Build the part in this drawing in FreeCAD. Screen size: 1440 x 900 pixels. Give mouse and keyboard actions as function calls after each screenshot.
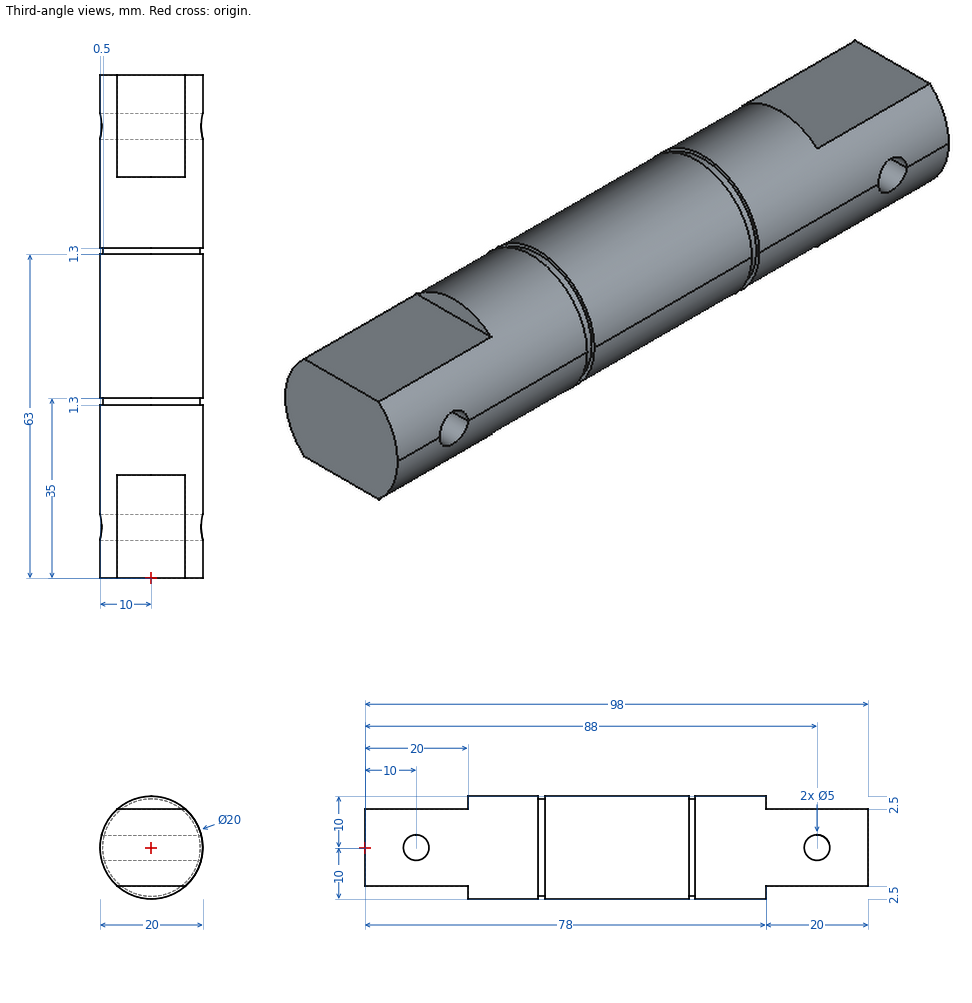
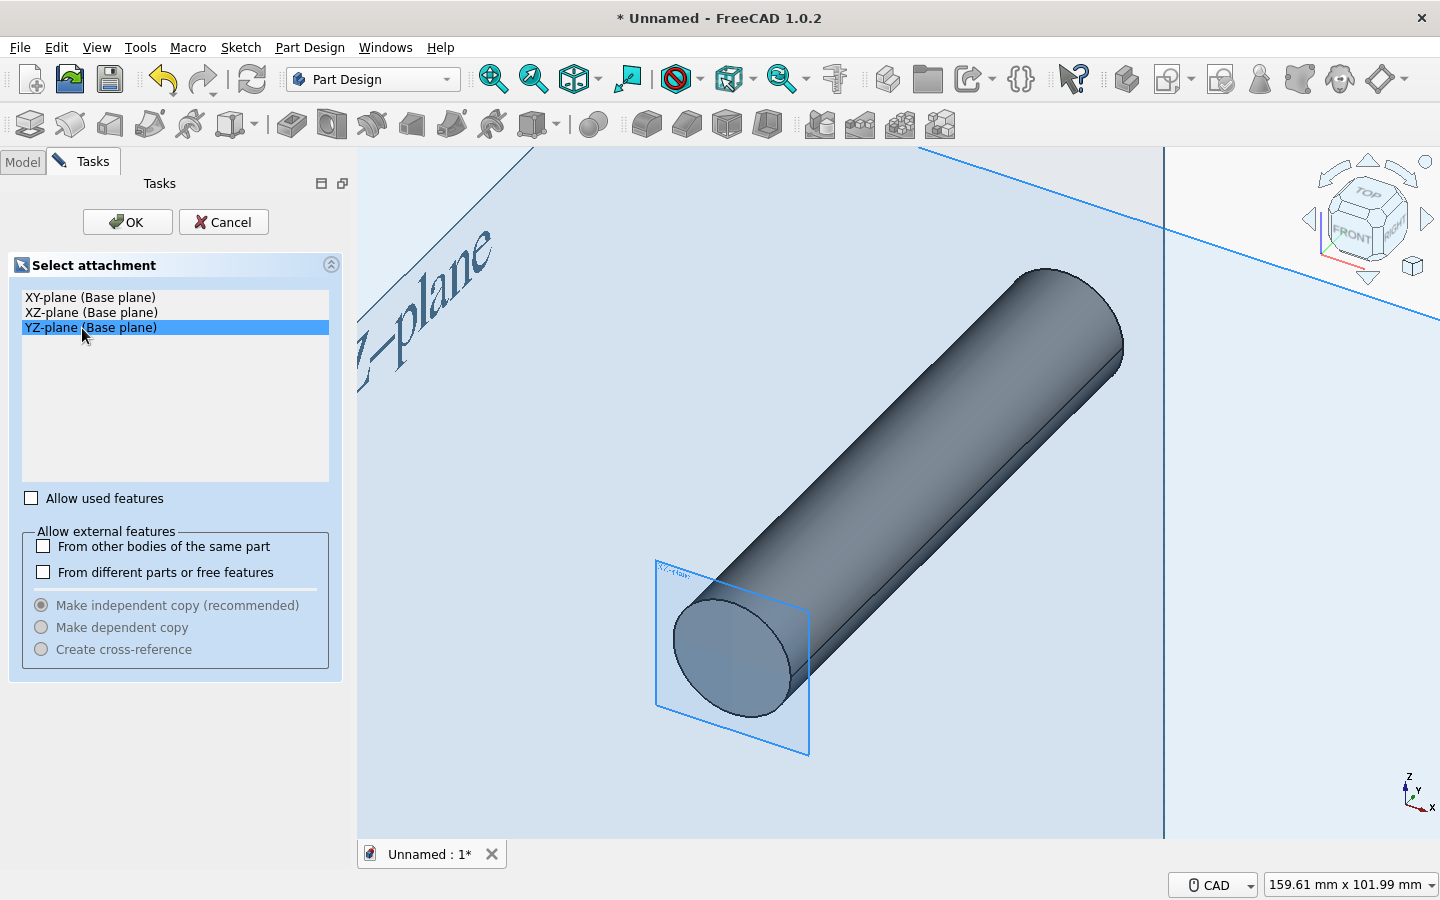
click(128, 222)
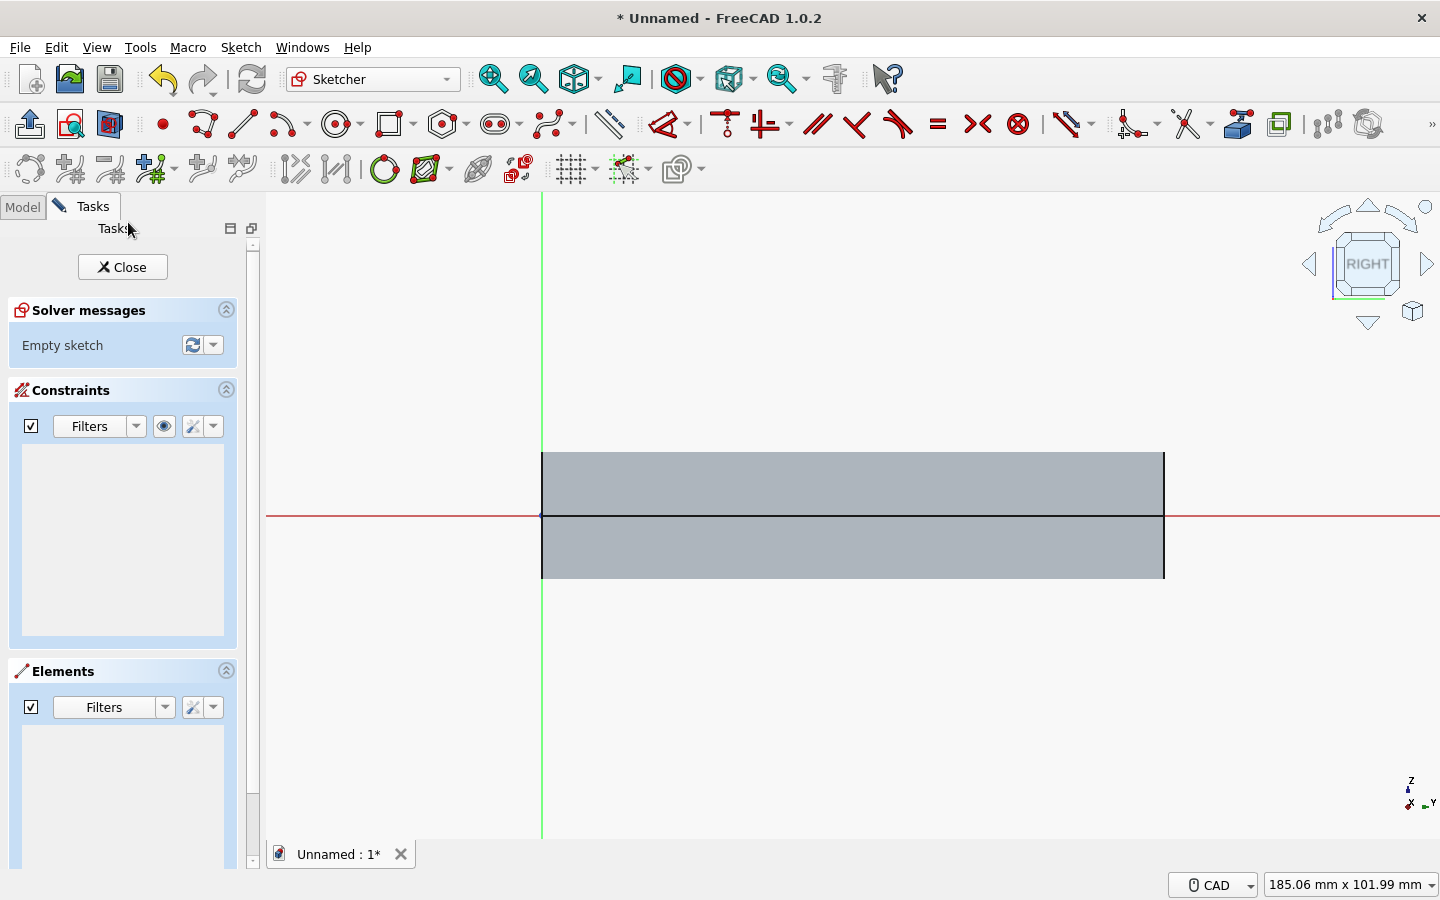
click(110, 124)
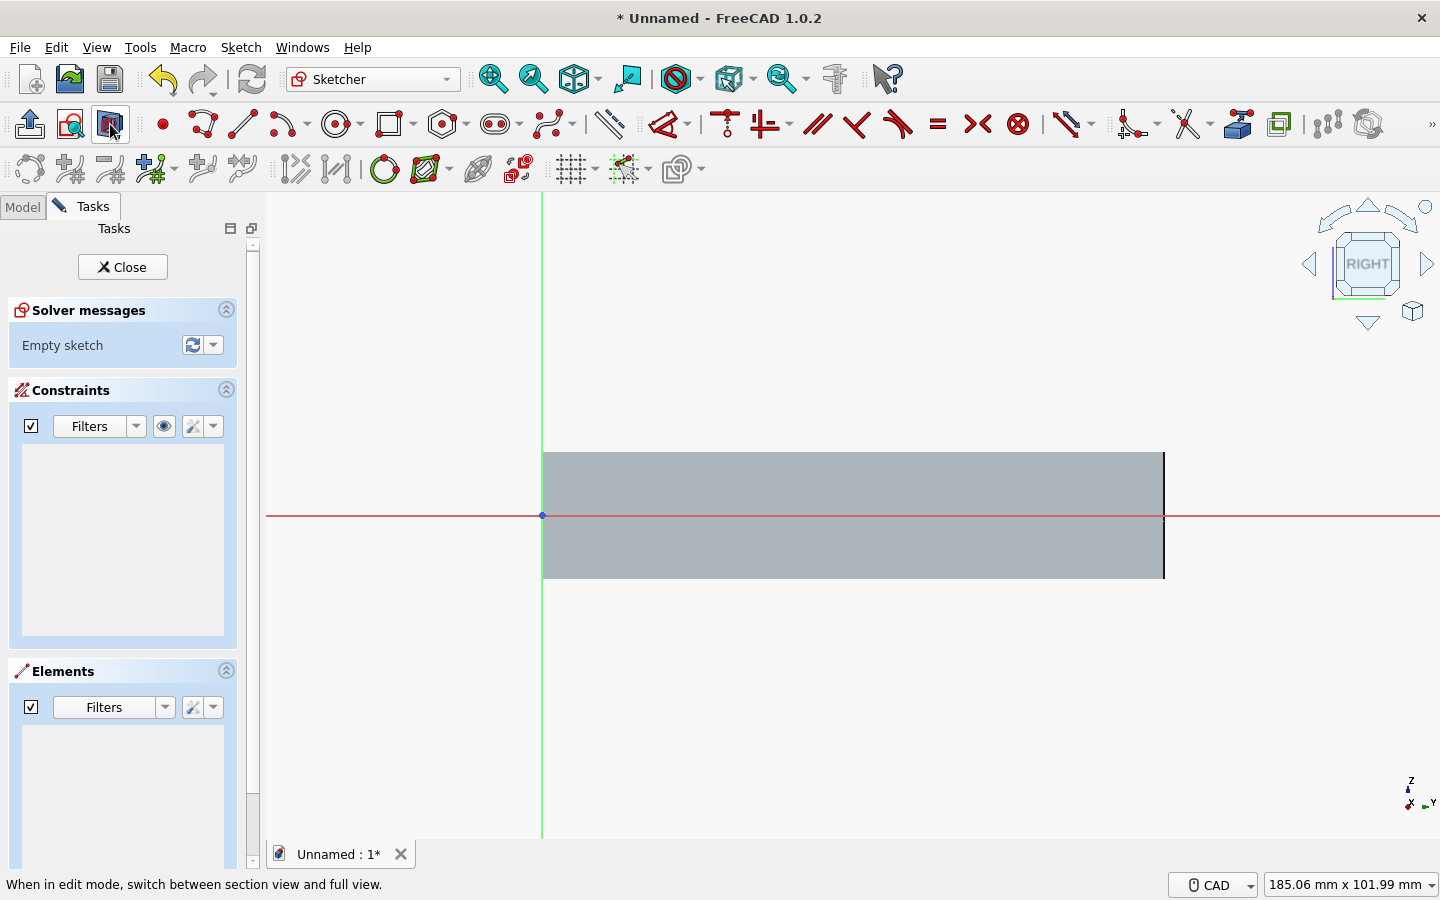
key(g)
key(r)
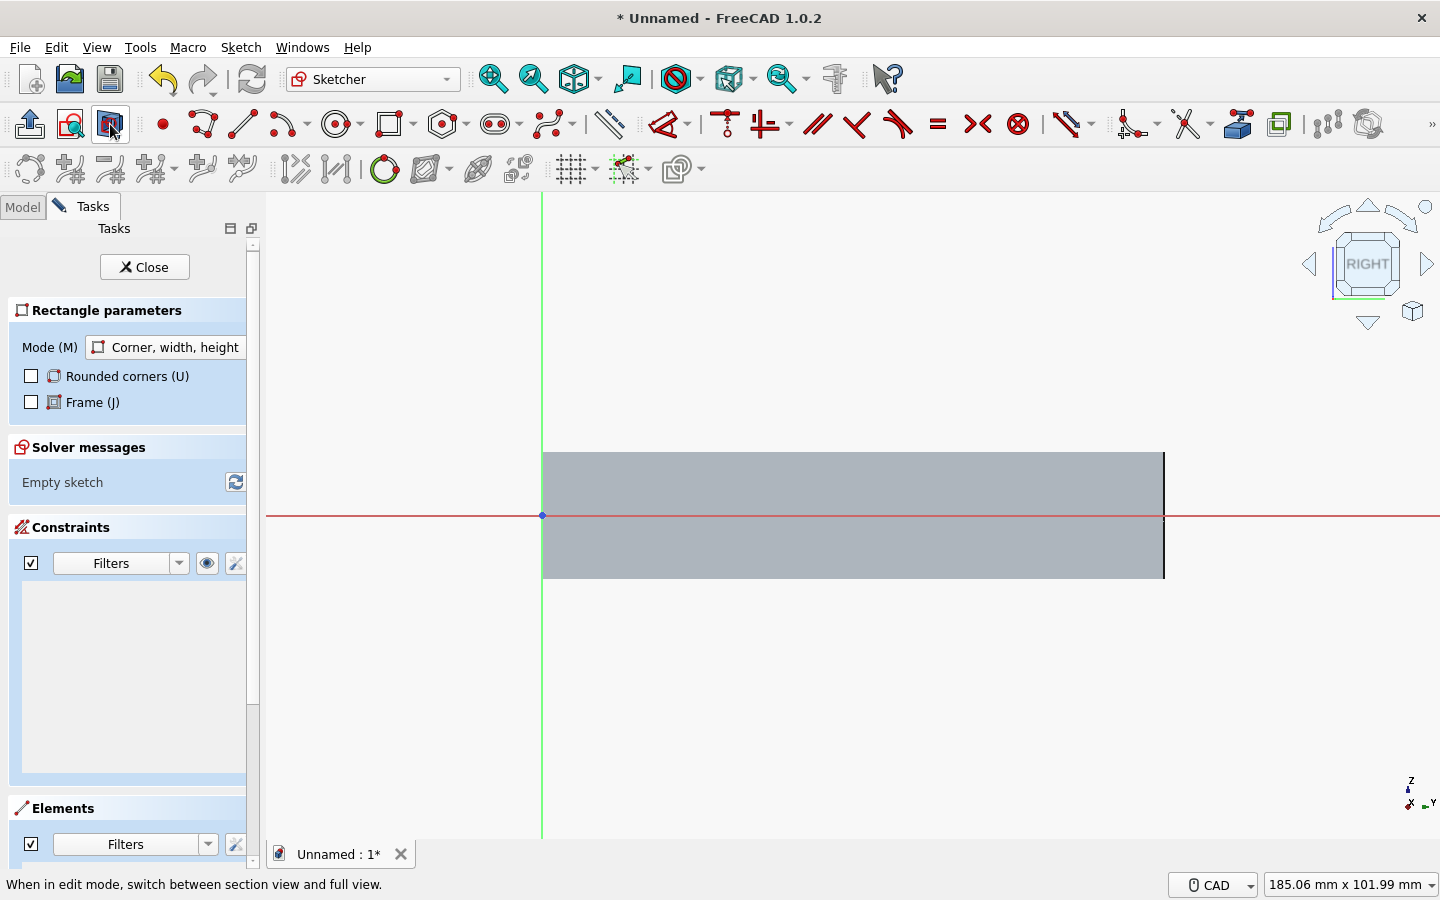
click(1037, 563)
move(1164, 579)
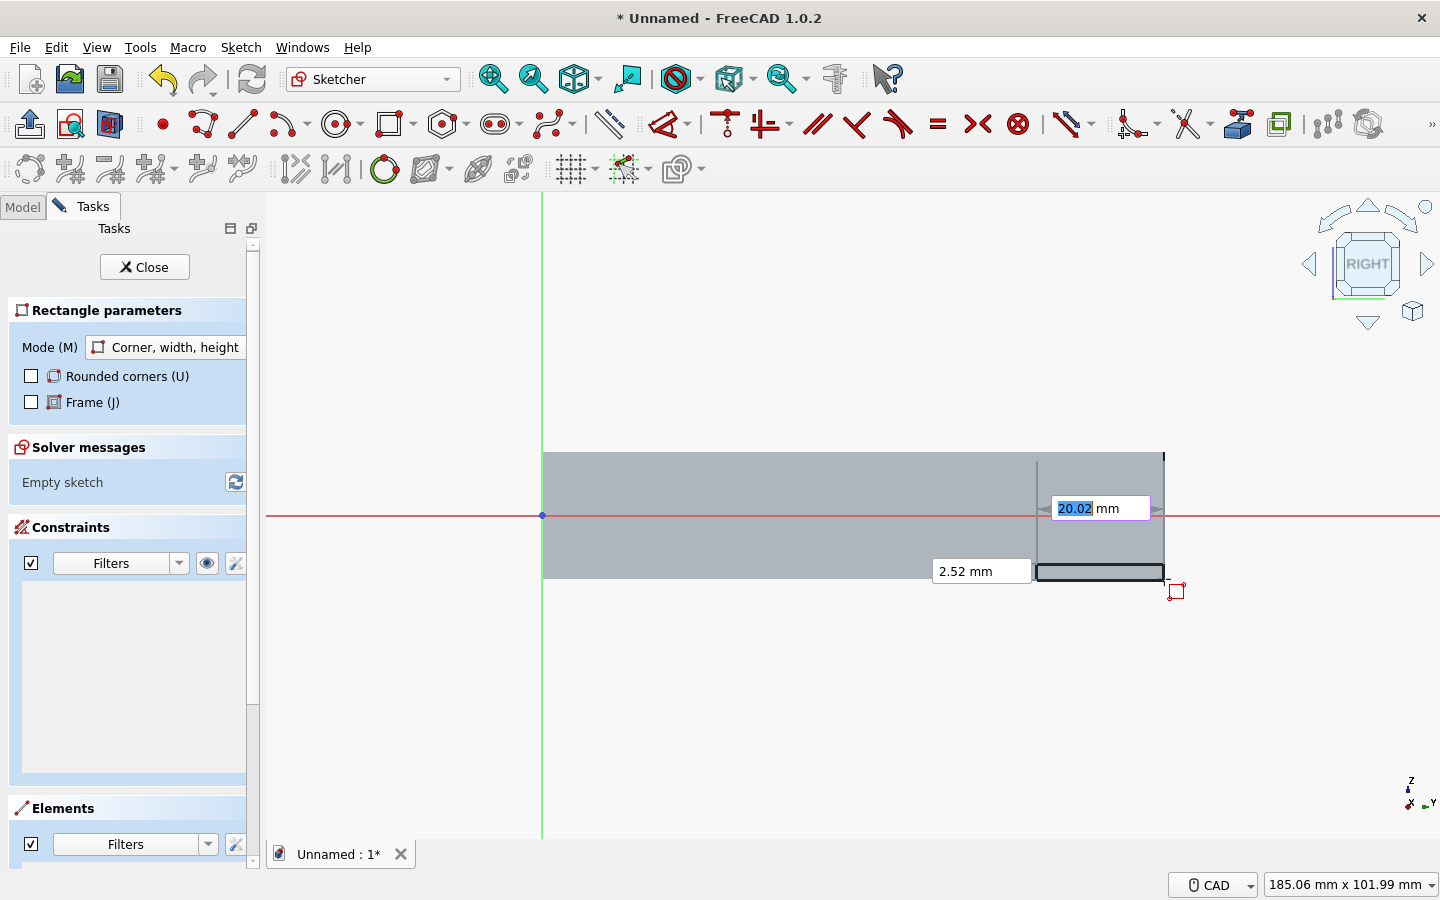
text(20)
key(Tab)
text(2.5)
key(Return)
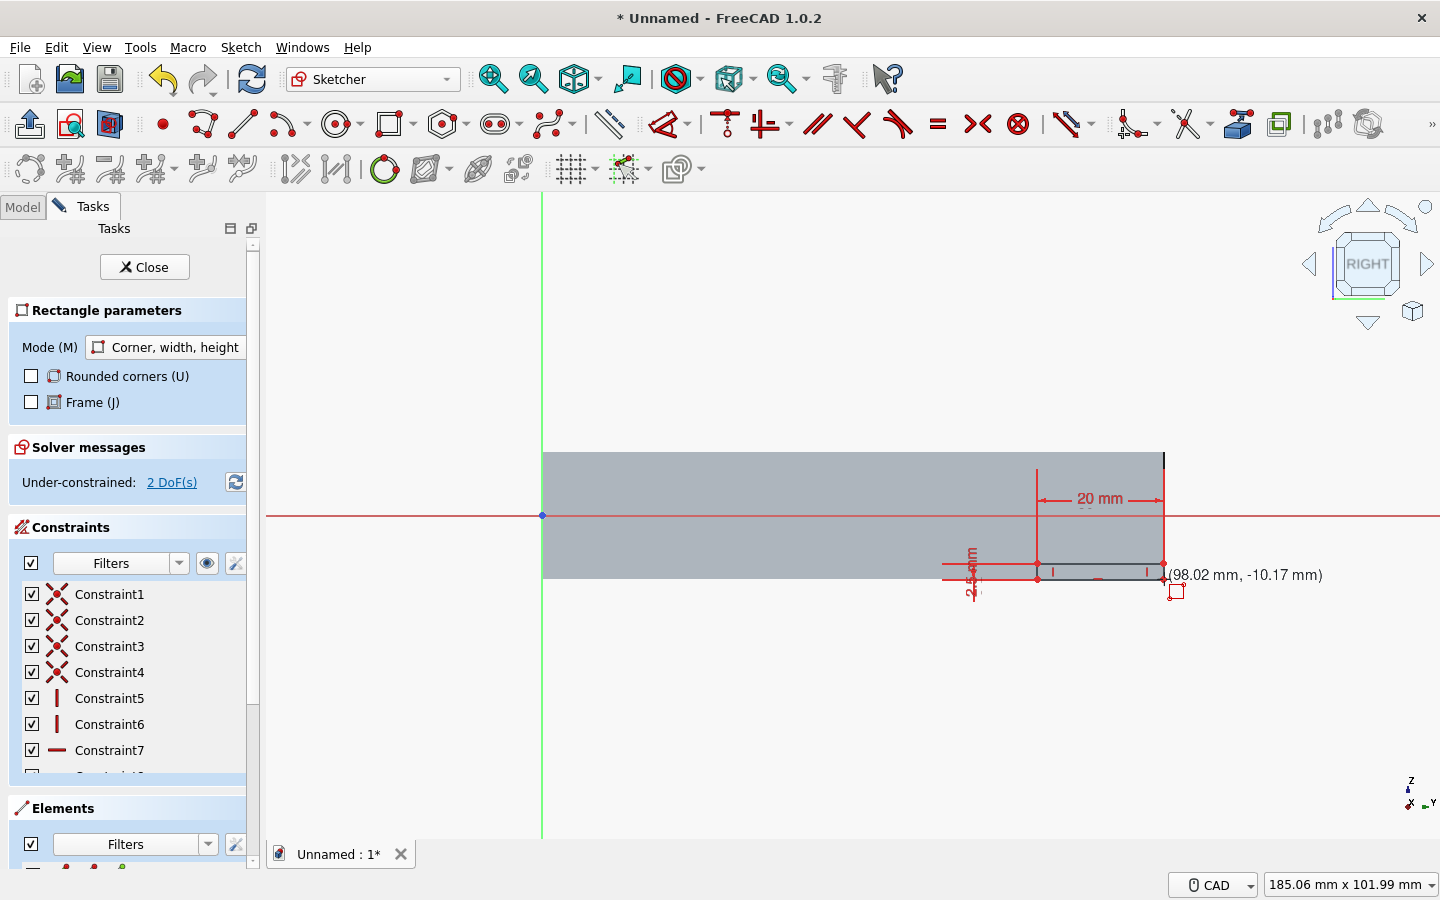
click(1037, 452)
move(1164, 468)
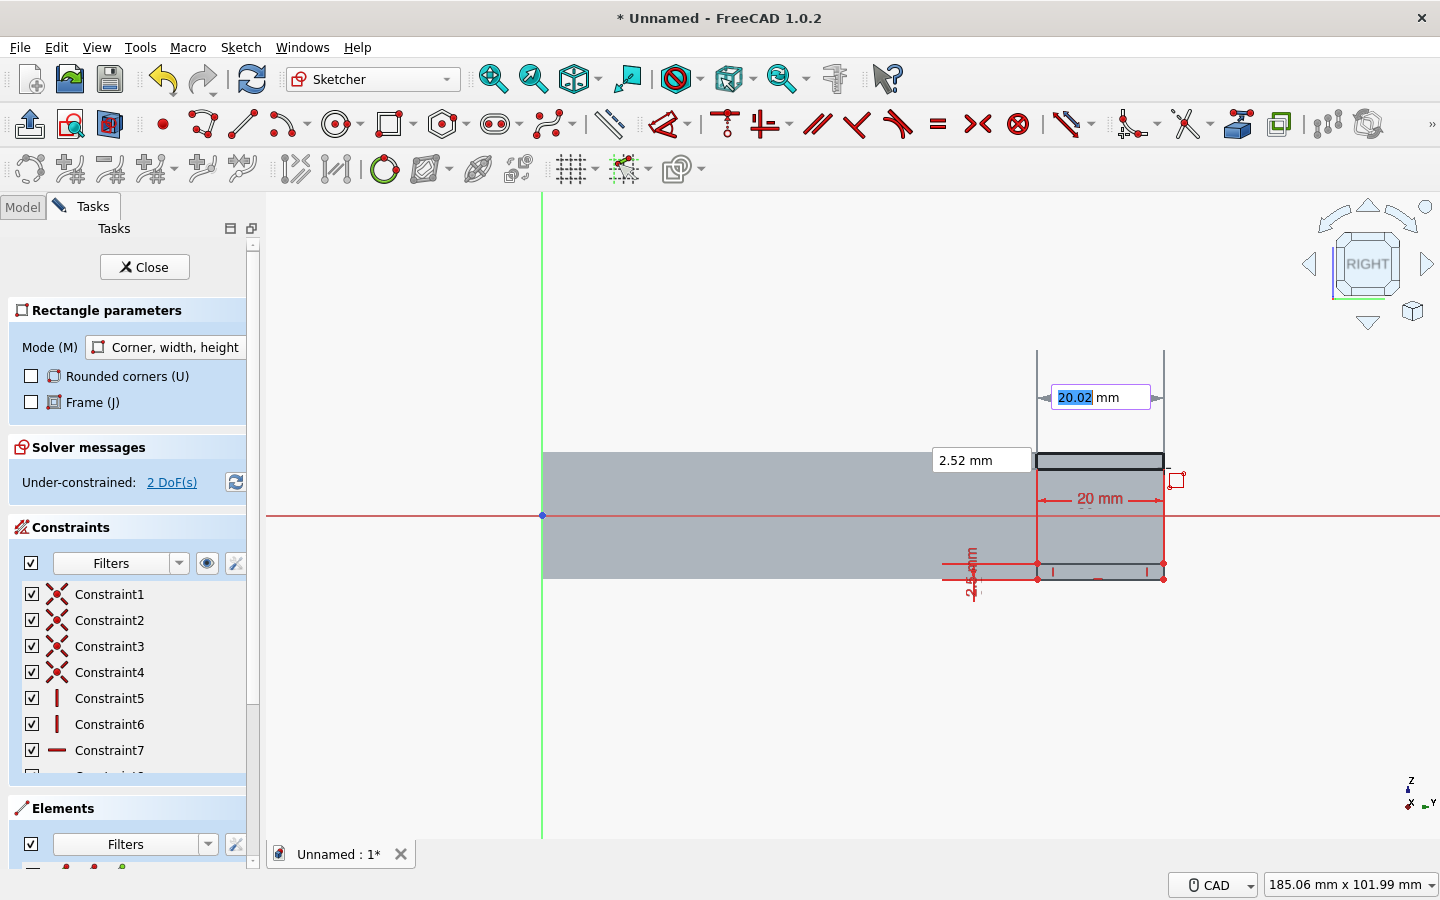
text(20)
key(Tab)
text(2.5)
key(Return)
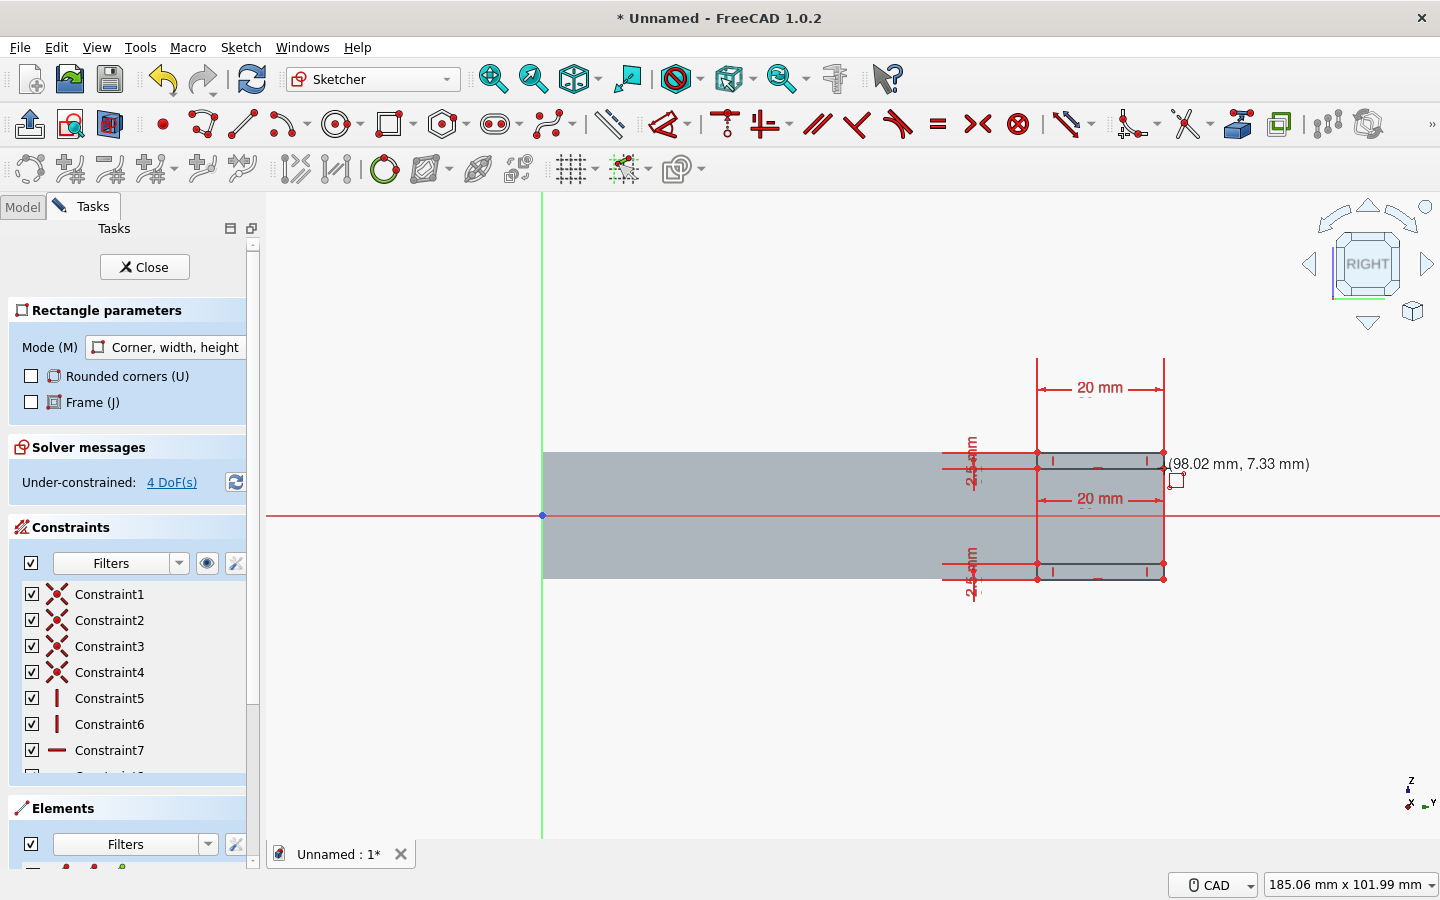
click(542, 452)
move(669, 468)